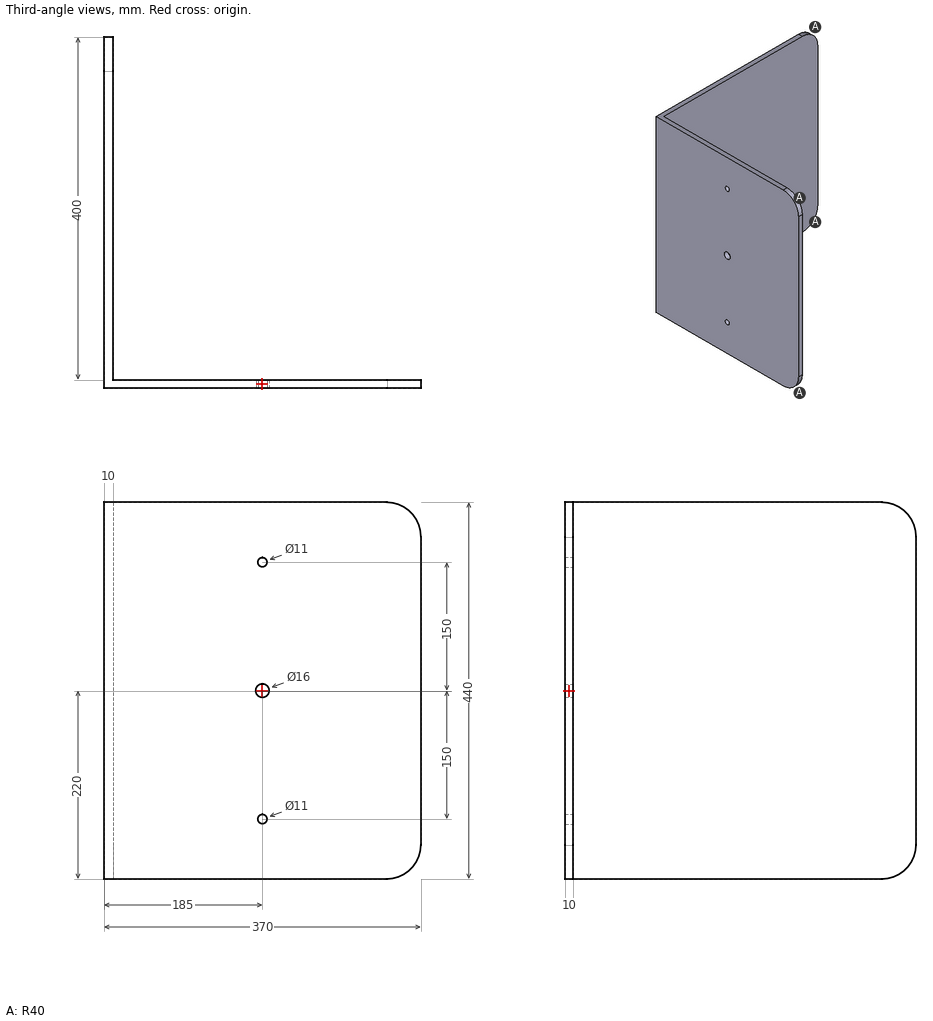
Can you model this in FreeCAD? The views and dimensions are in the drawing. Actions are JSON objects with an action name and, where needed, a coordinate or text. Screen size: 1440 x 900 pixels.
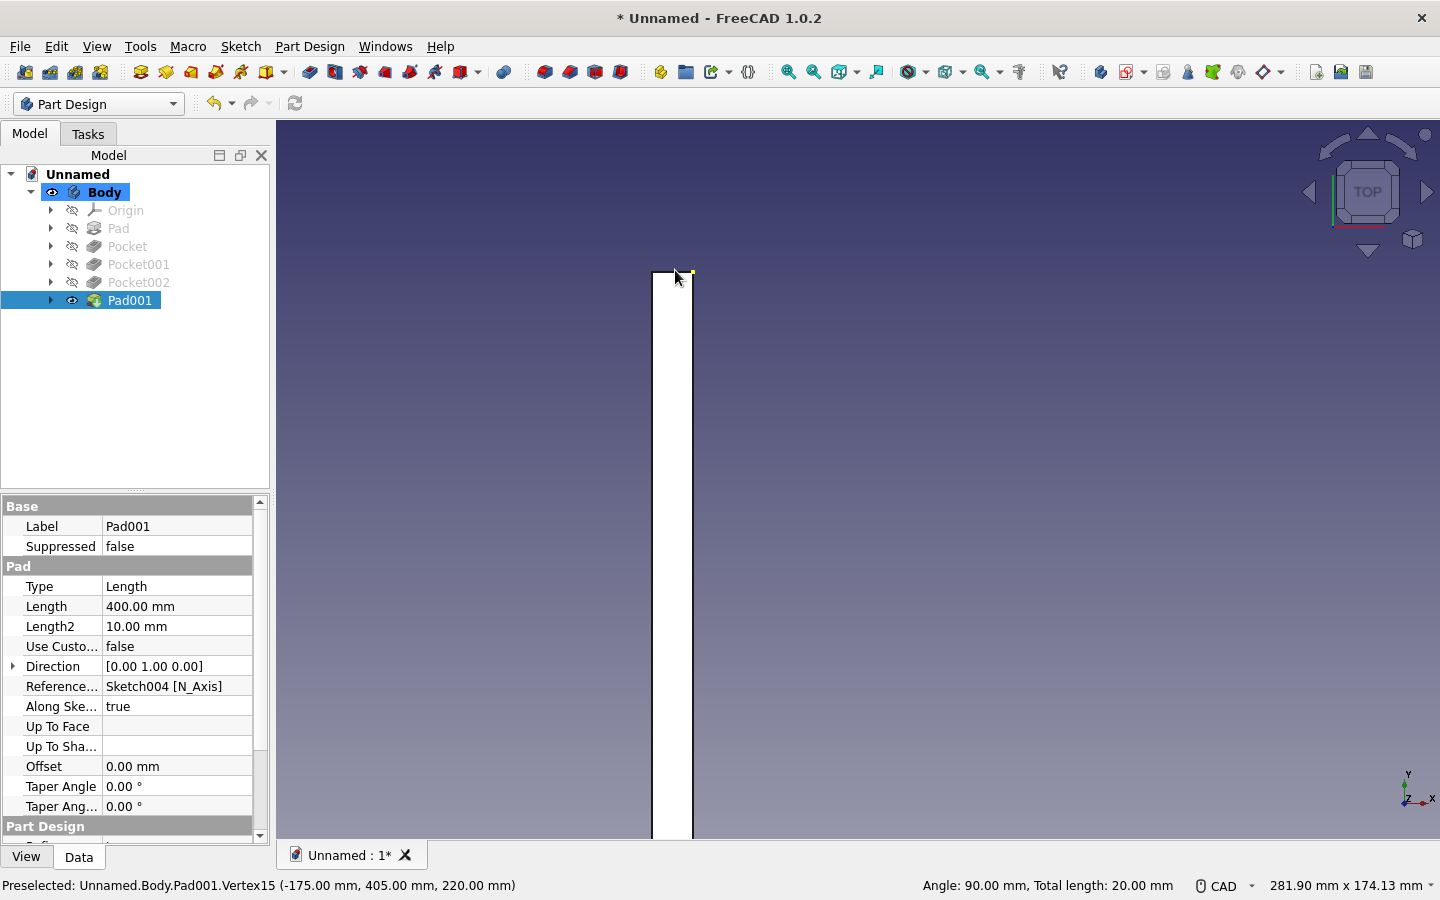
{"action": "left_click", "coordinate": [673, 271], "text": "ctrl"}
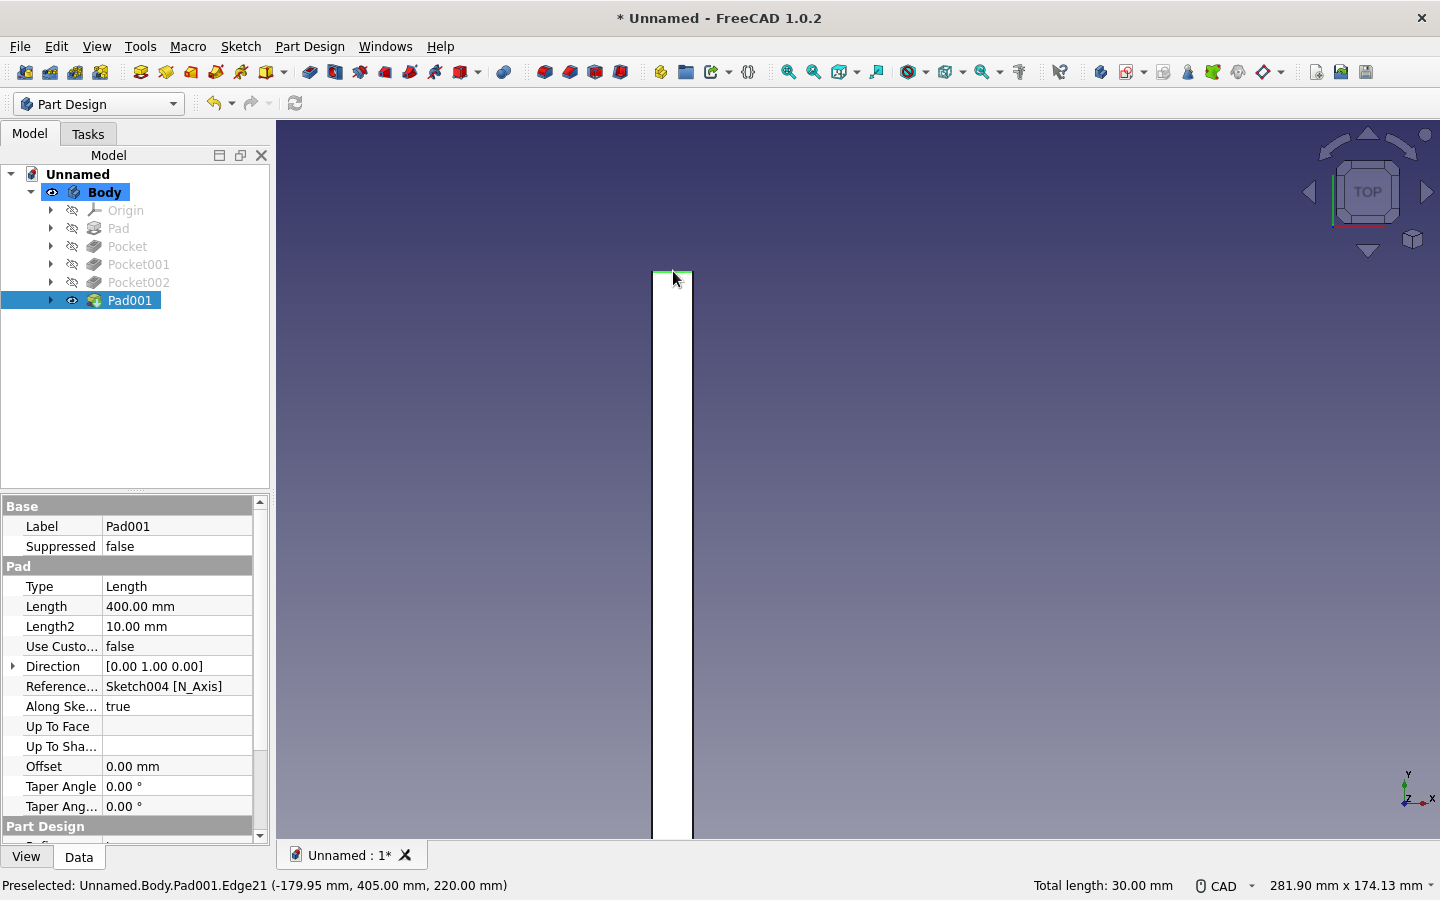
{"action": "left_click", "coordinate": [789, 72]}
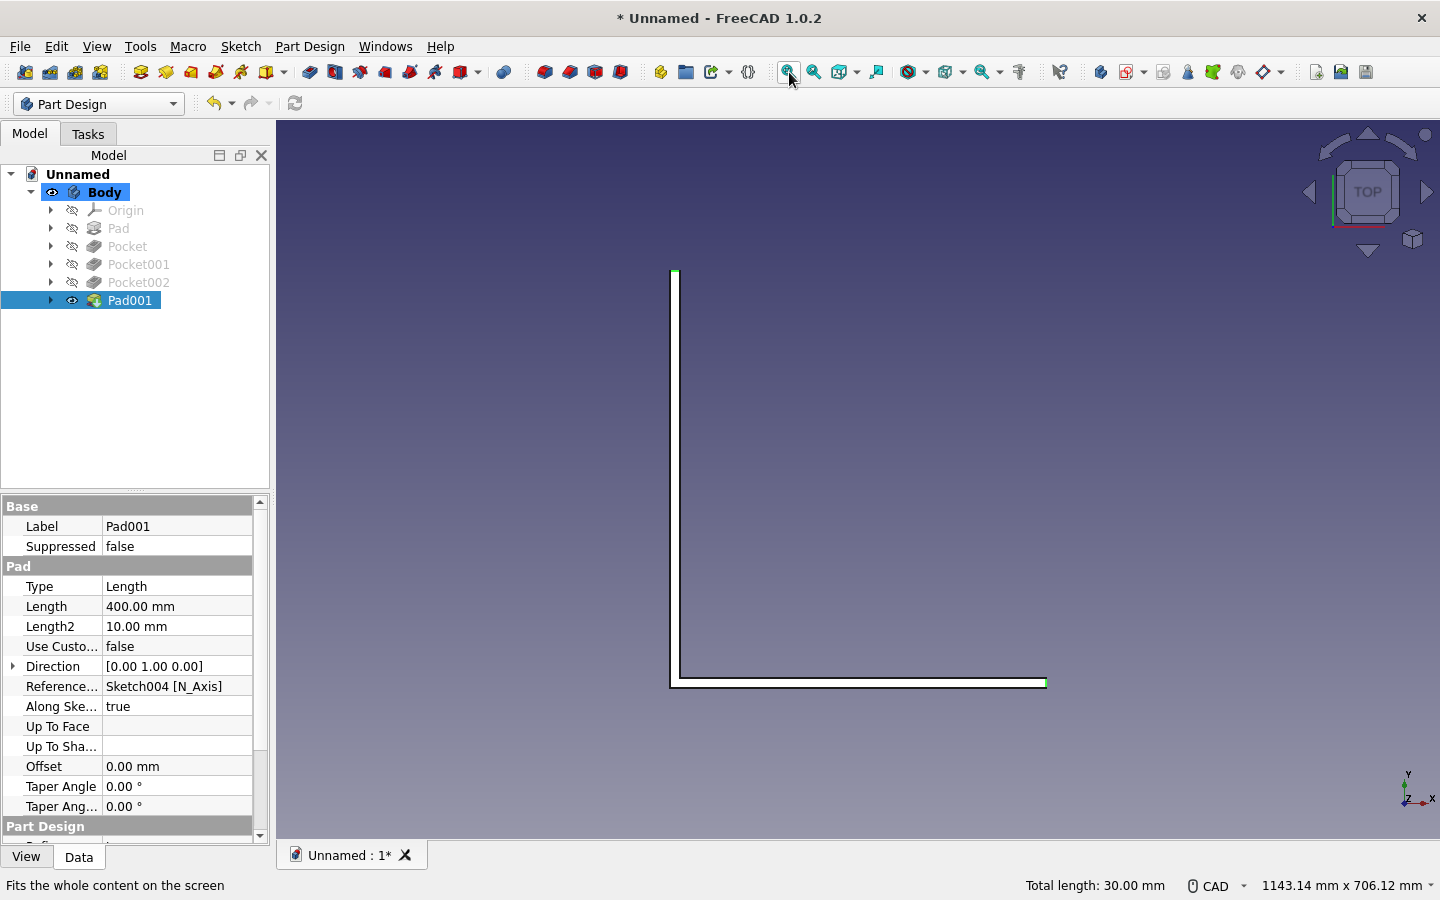
{"action": "key", "text": "1"}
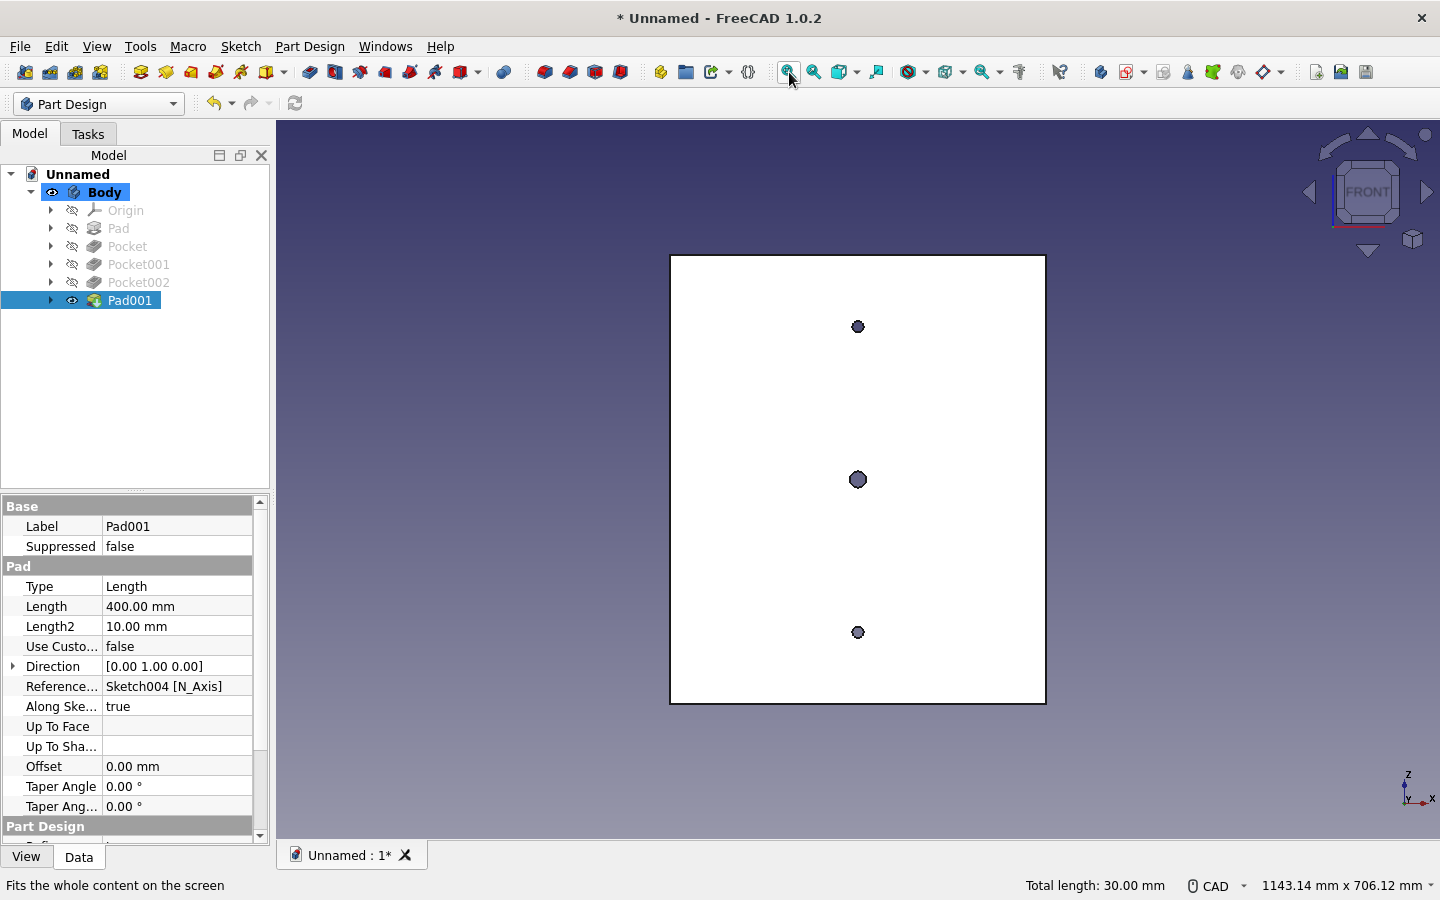
{"action": "scroll", "coordinate": [1046, 703], "scroll_direction": "up", "scroll_amount": 7}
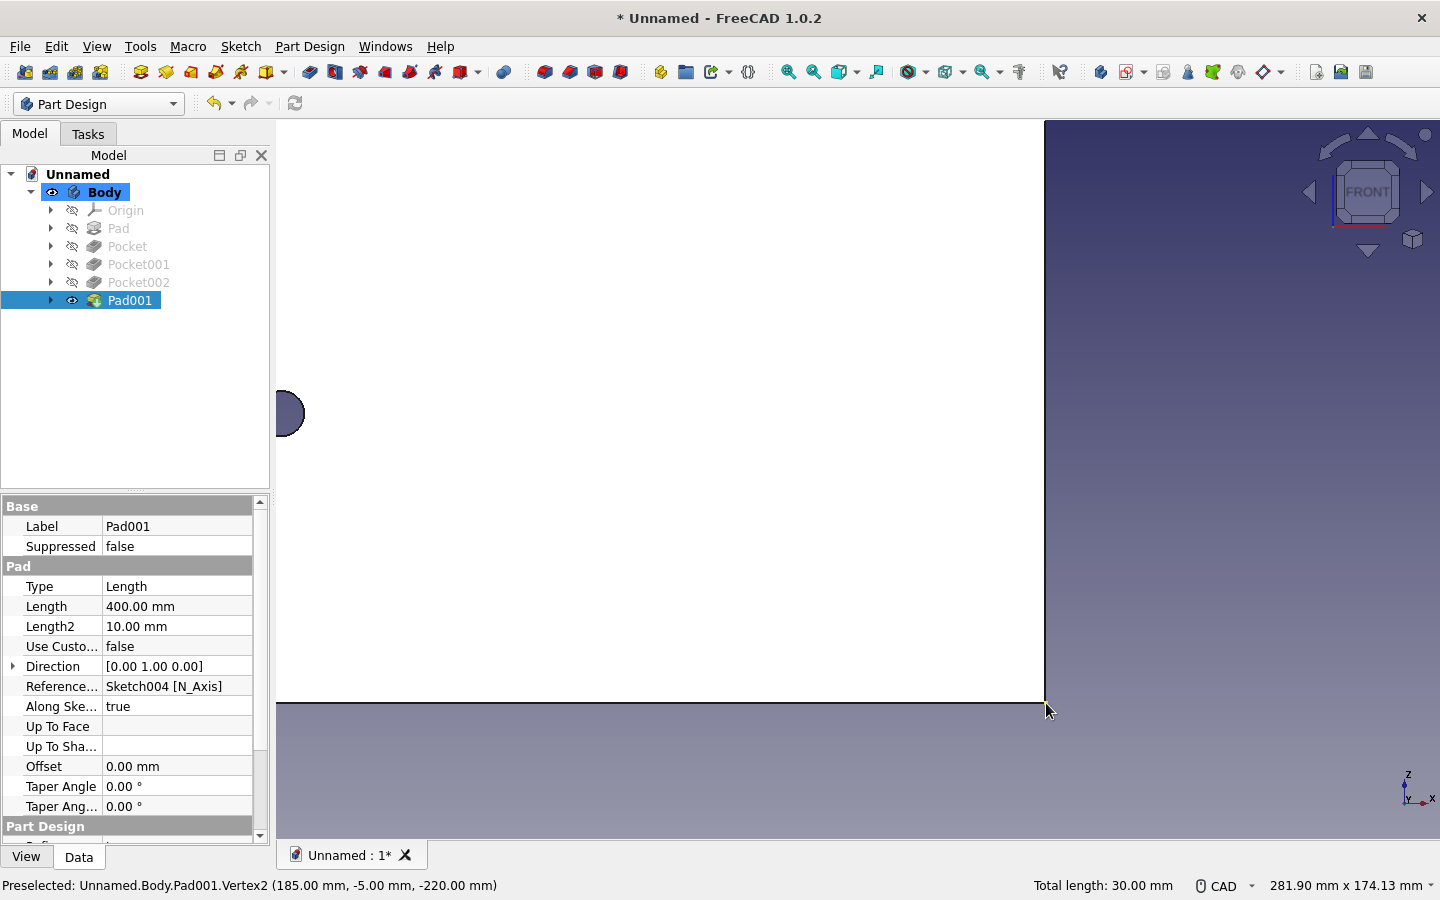
{"action": "left_click", "coordinate": [789, 72]}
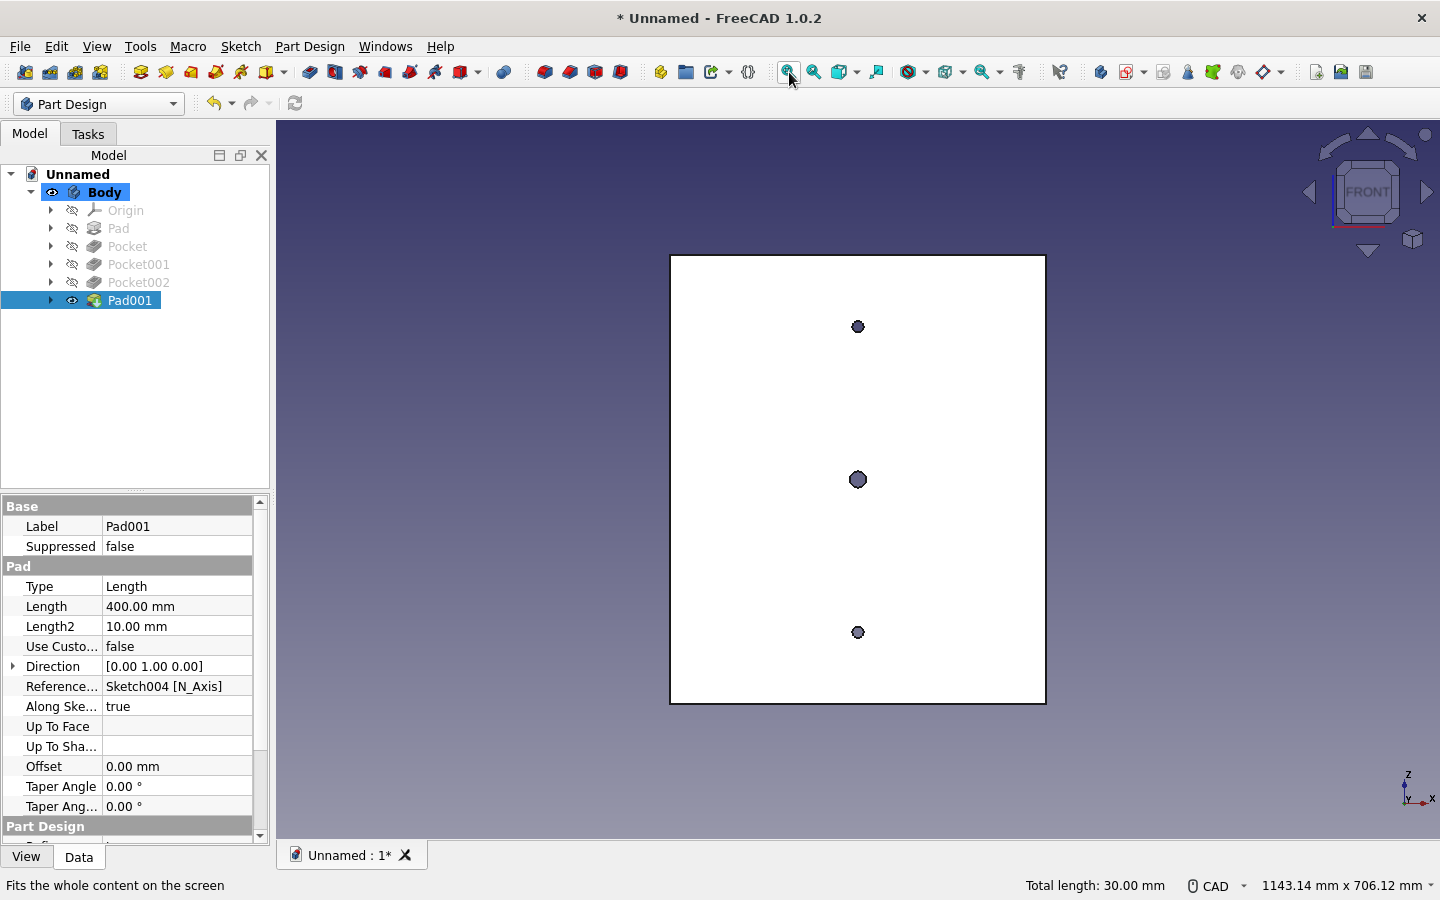
{"action": "key", "text": "3"}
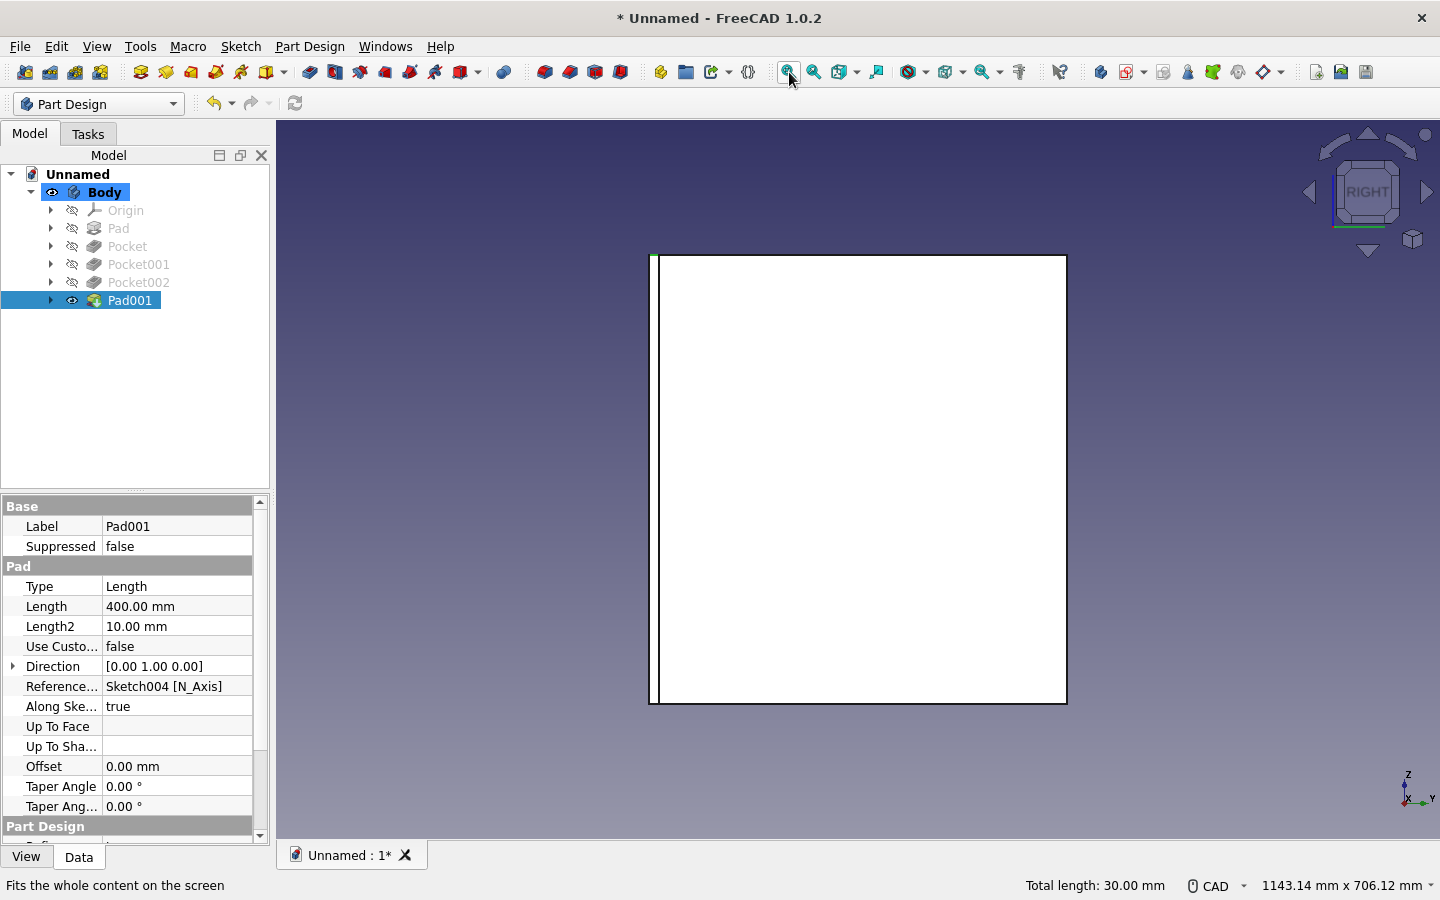
{"action": "scroll", "coordinate": [654, 703], "scroll_direction": "up", "scroll_amount": 7}